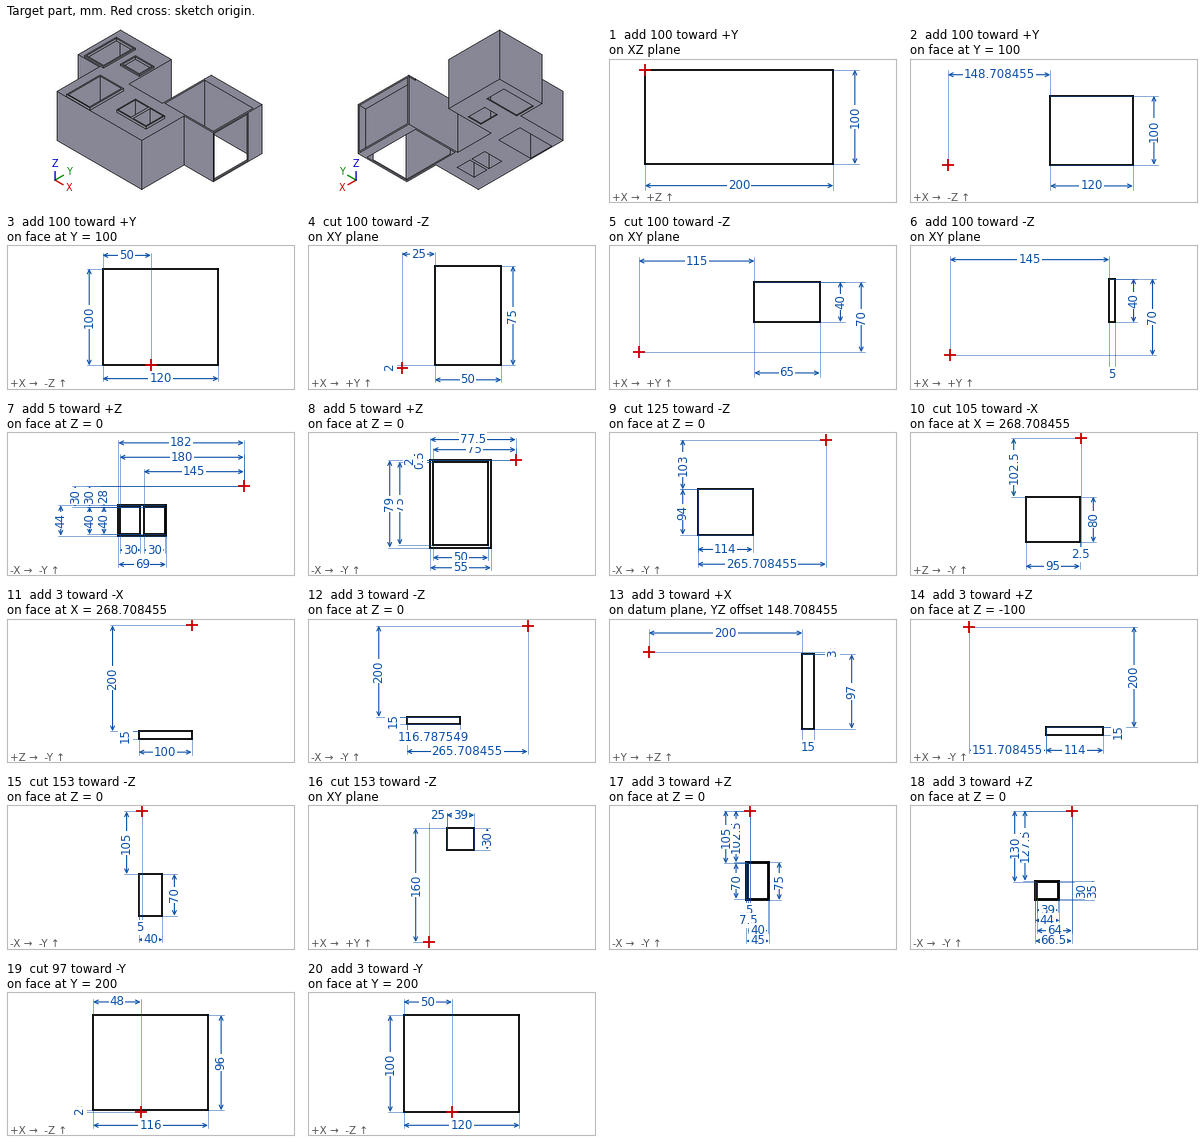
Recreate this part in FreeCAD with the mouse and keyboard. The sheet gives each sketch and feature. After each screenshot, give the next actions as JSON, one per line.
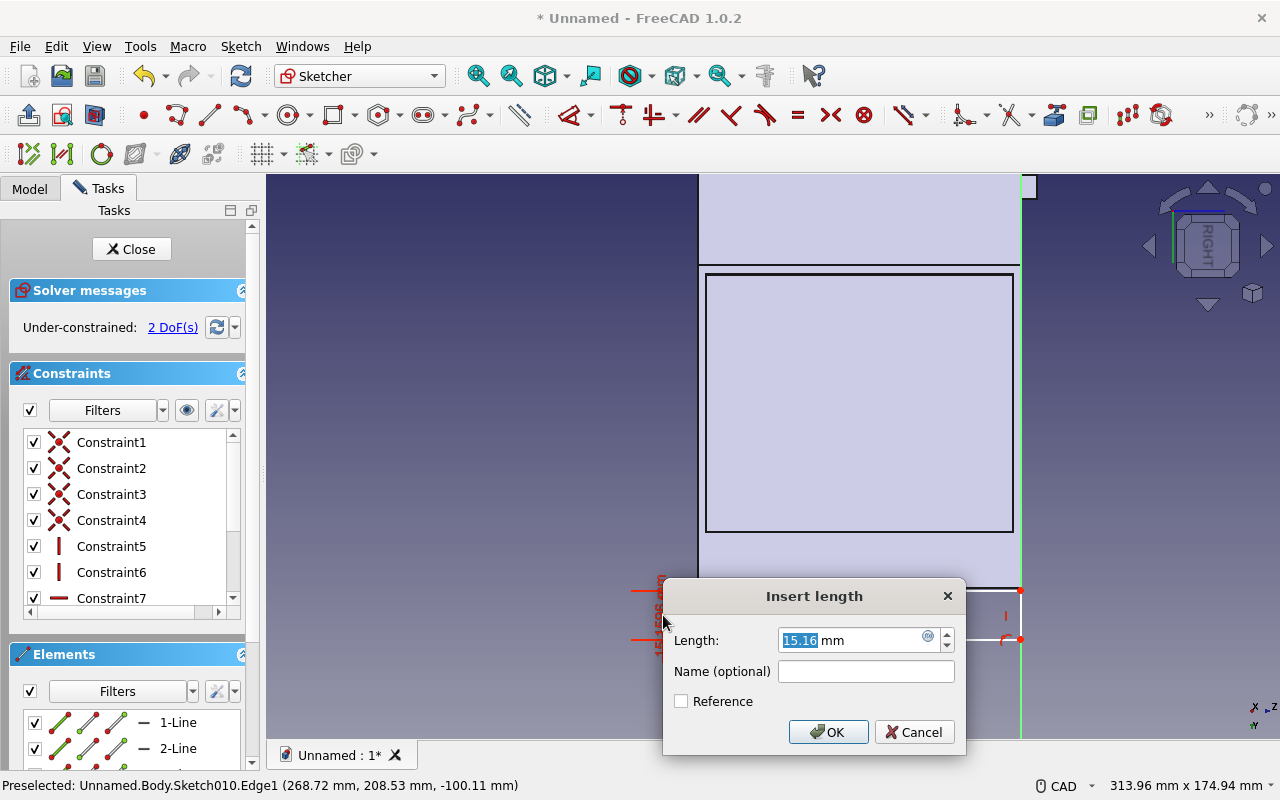
{"action": "type", "text": "15"}
{"action": "key", "text": "Return"}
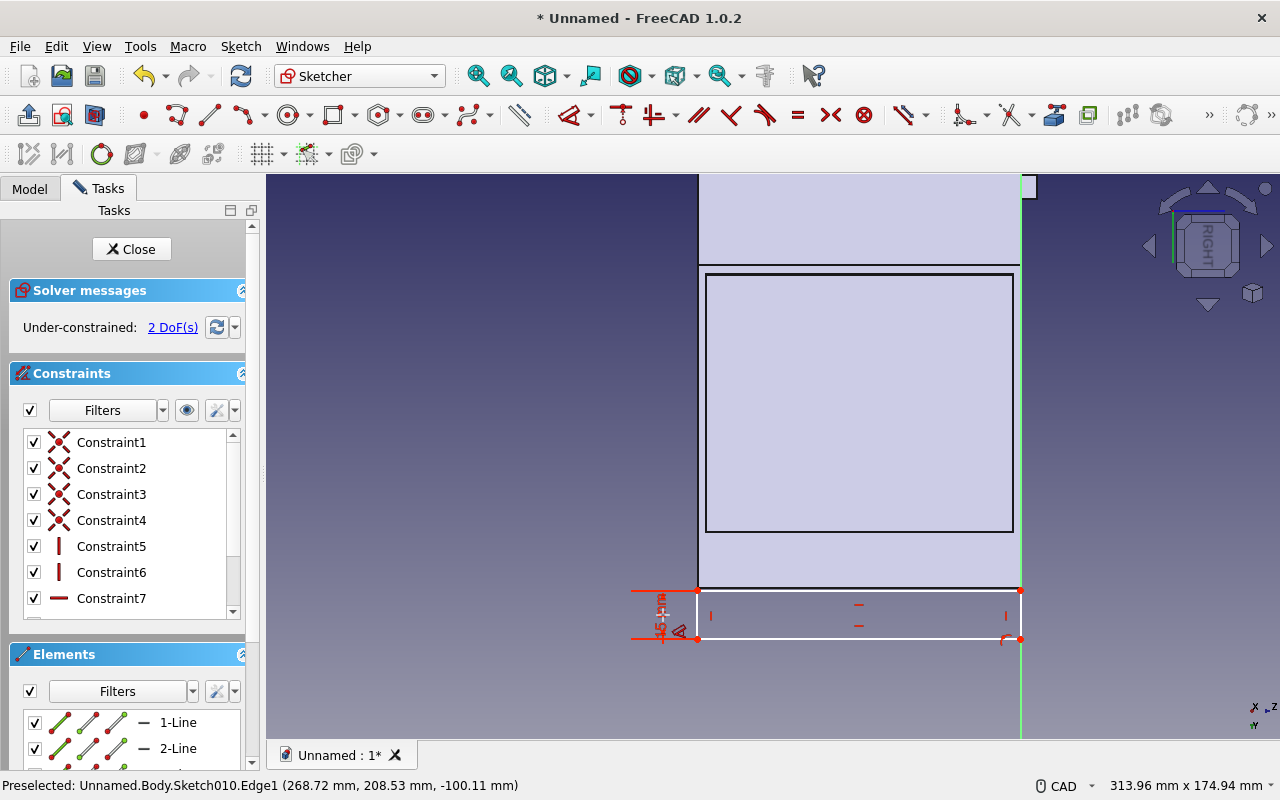
{"action": "left_click", "coordinate": [794, 639]}
{"action": "left_click", "coordinate": [859, 673]}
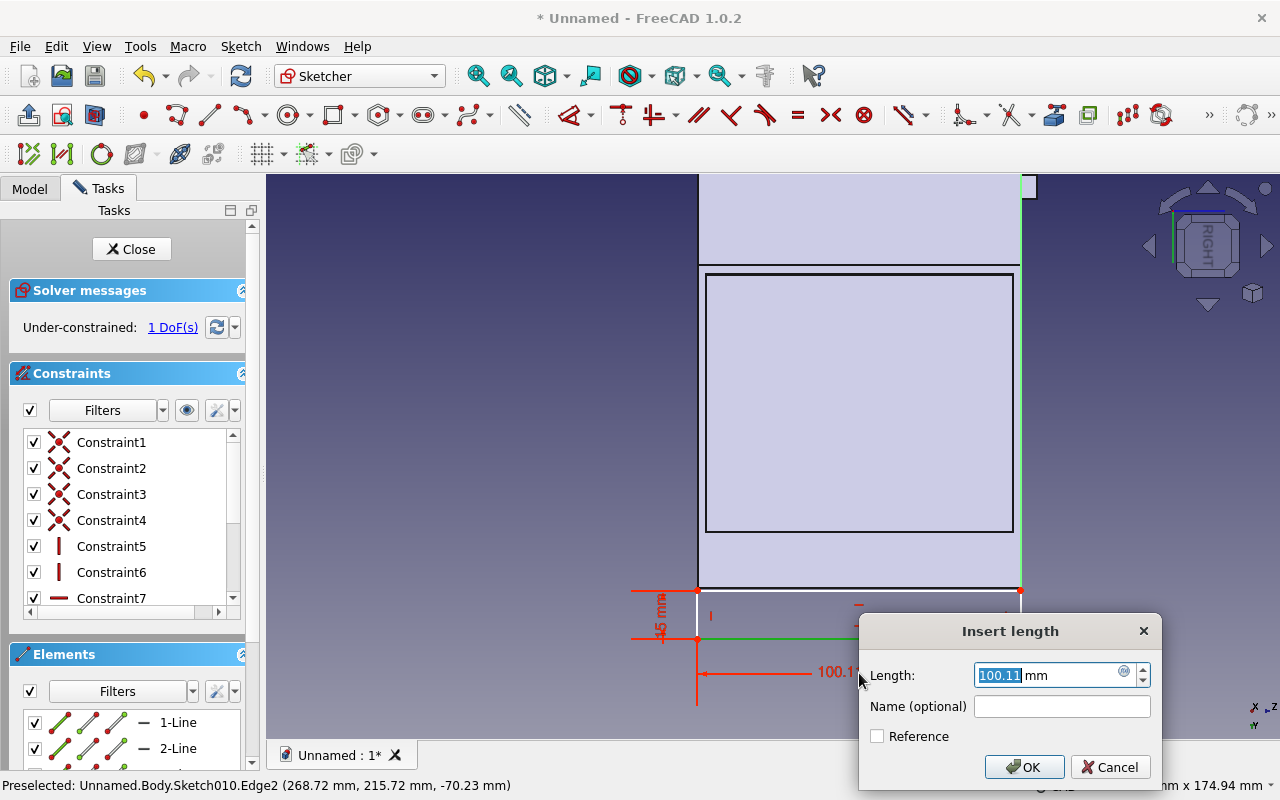
{"action": "type", "text": "100"}
{"action": "key", "text": "Return"}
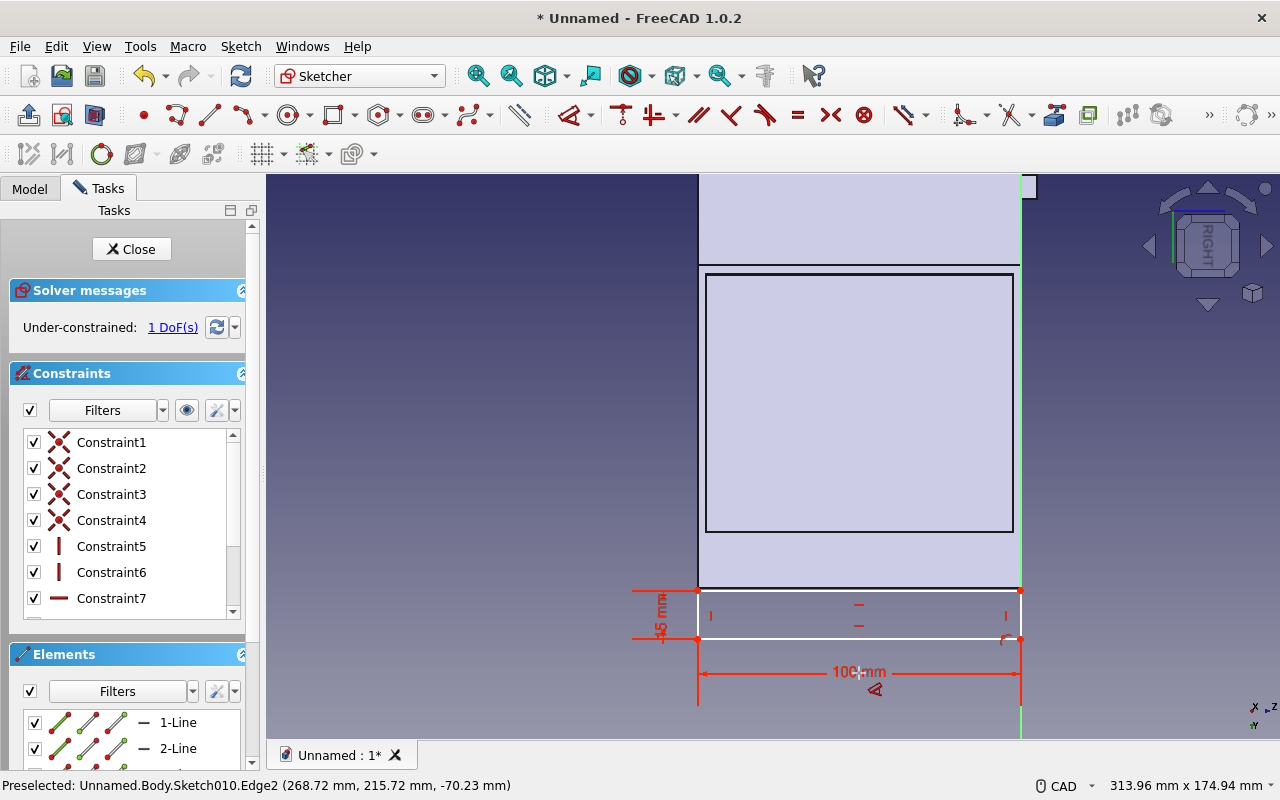
{"action": "left_click", "coordinate": [698, 591]}
{"action": "left_click", "coordinate": [1055, 396]}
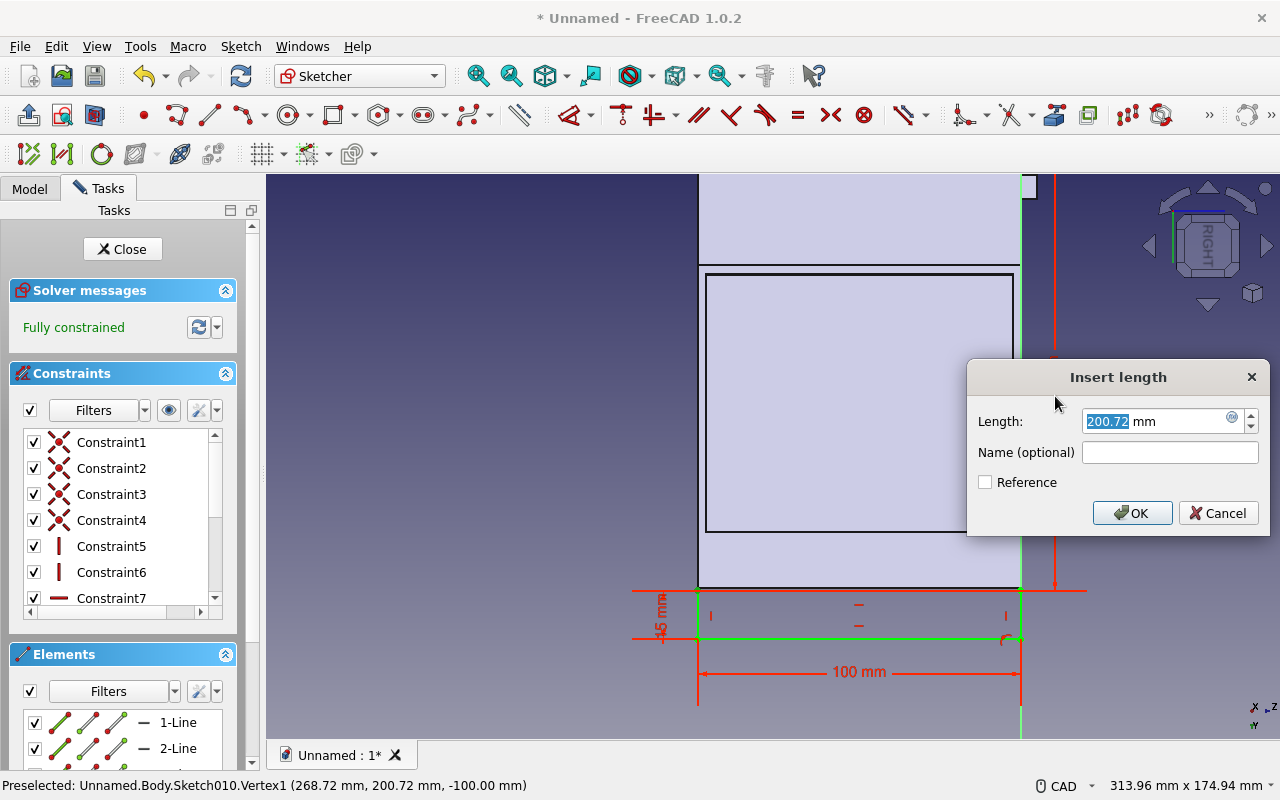
{"action": "type", "text": "200"}
{"action": "key", "text": "Return"}
{"action": "key", "text": "Escape"}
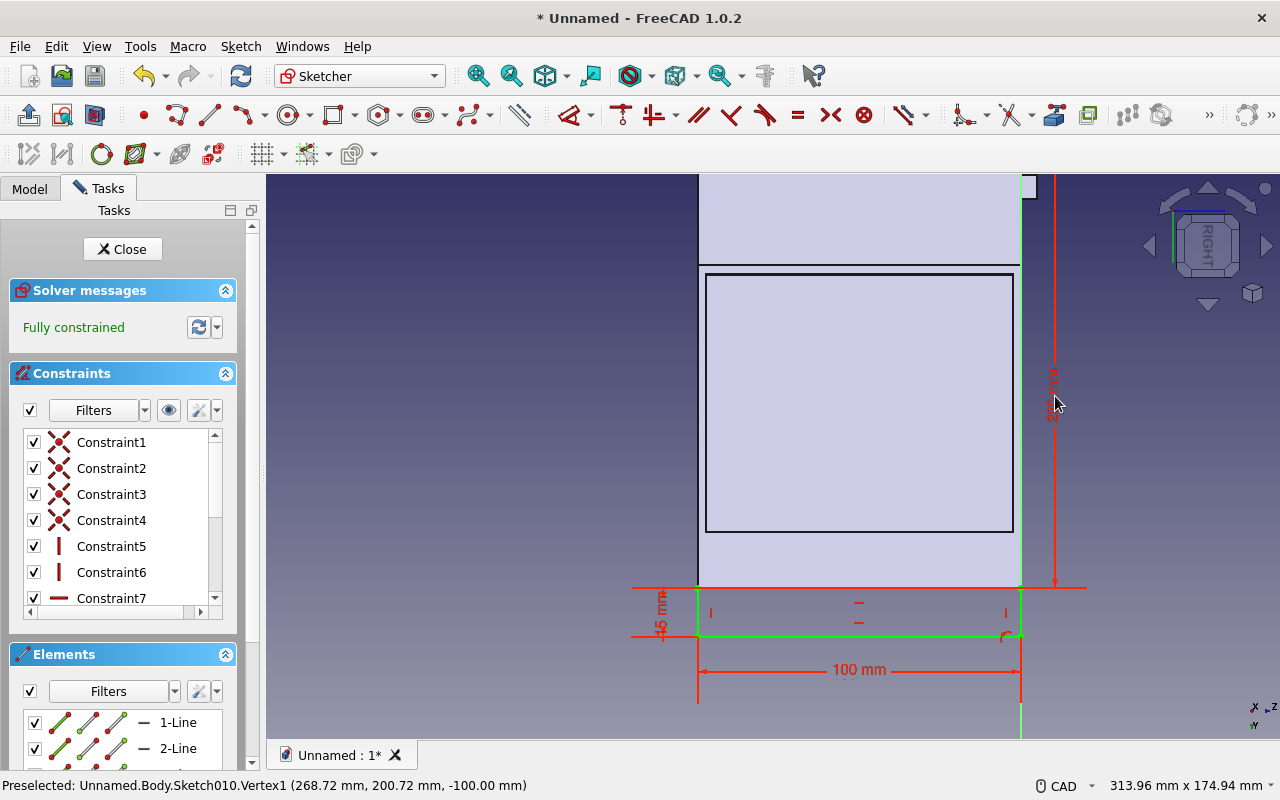
{"action": "left_click", "coordinate": [123, 249]}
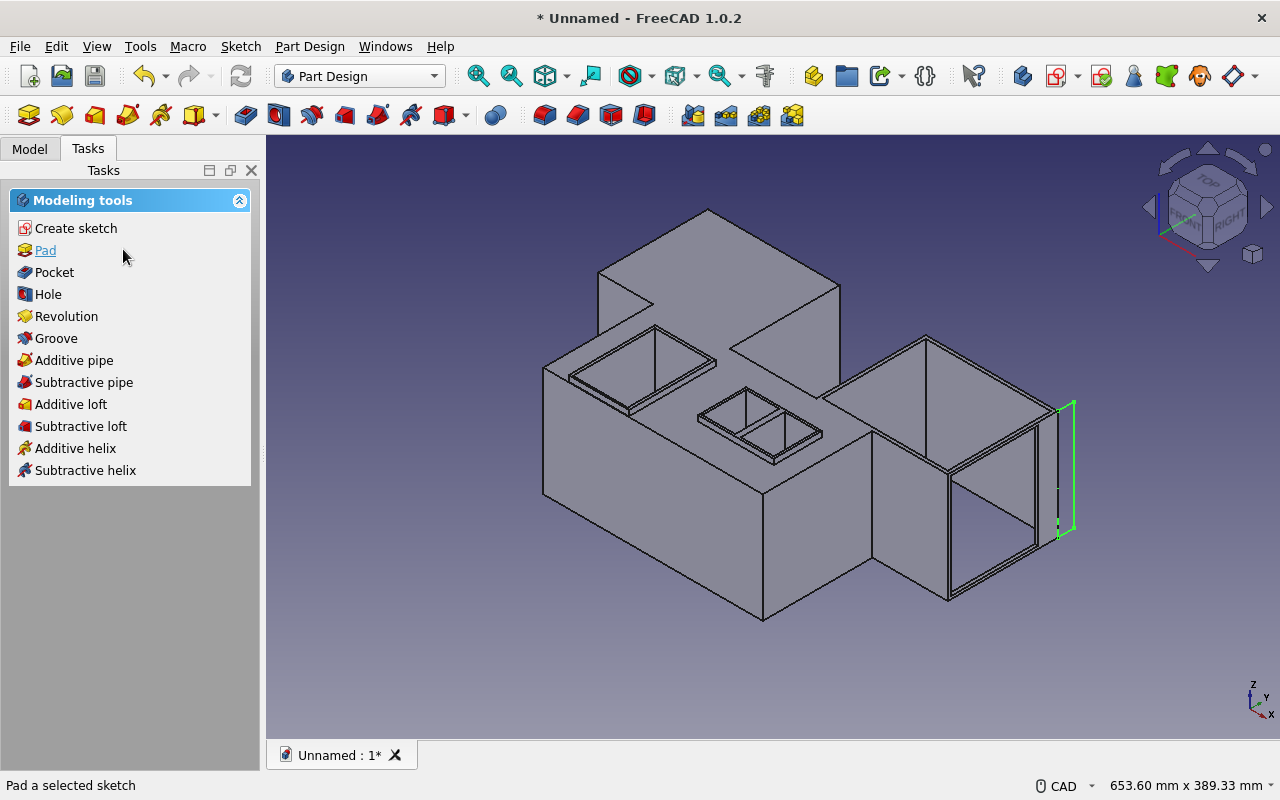
{"action": "left_click", "coordinate": [29, 116]}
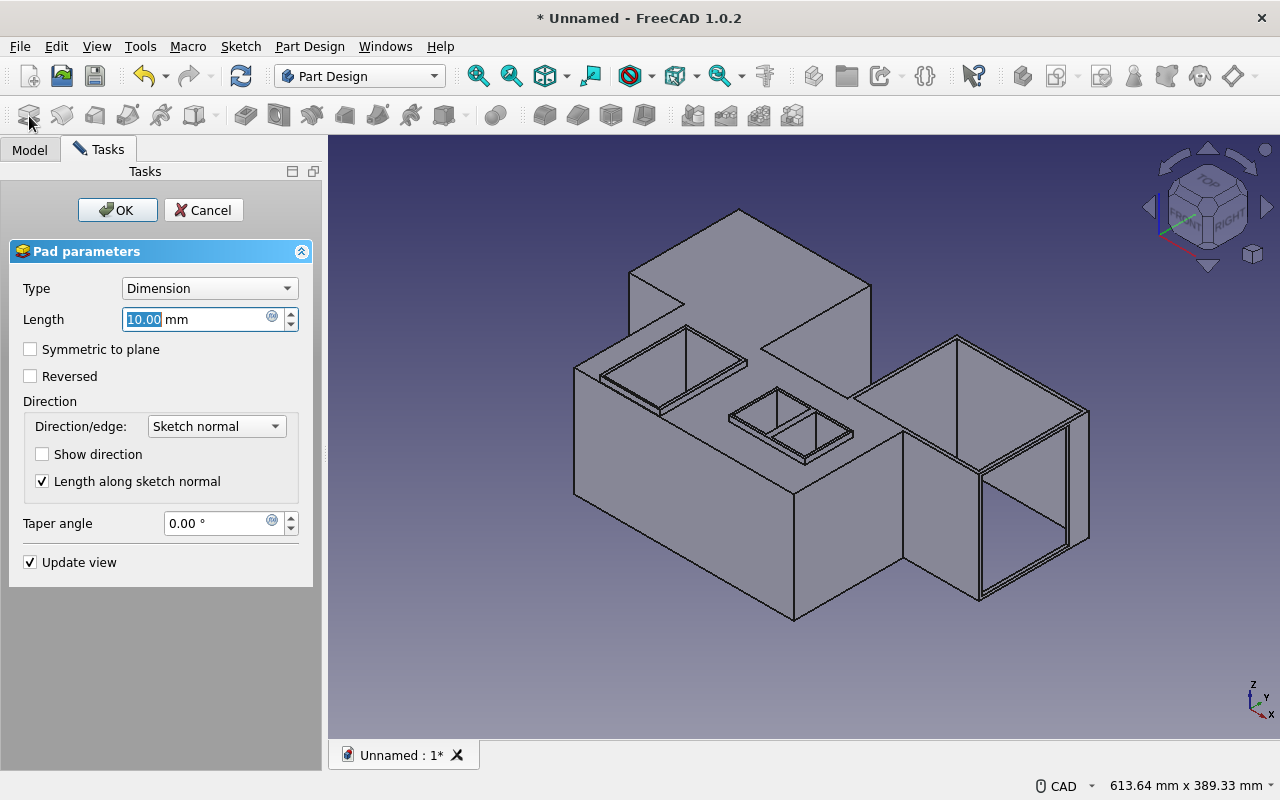
{"action": "type", "text": "3"}
{"action": "key", "text": "Tab"}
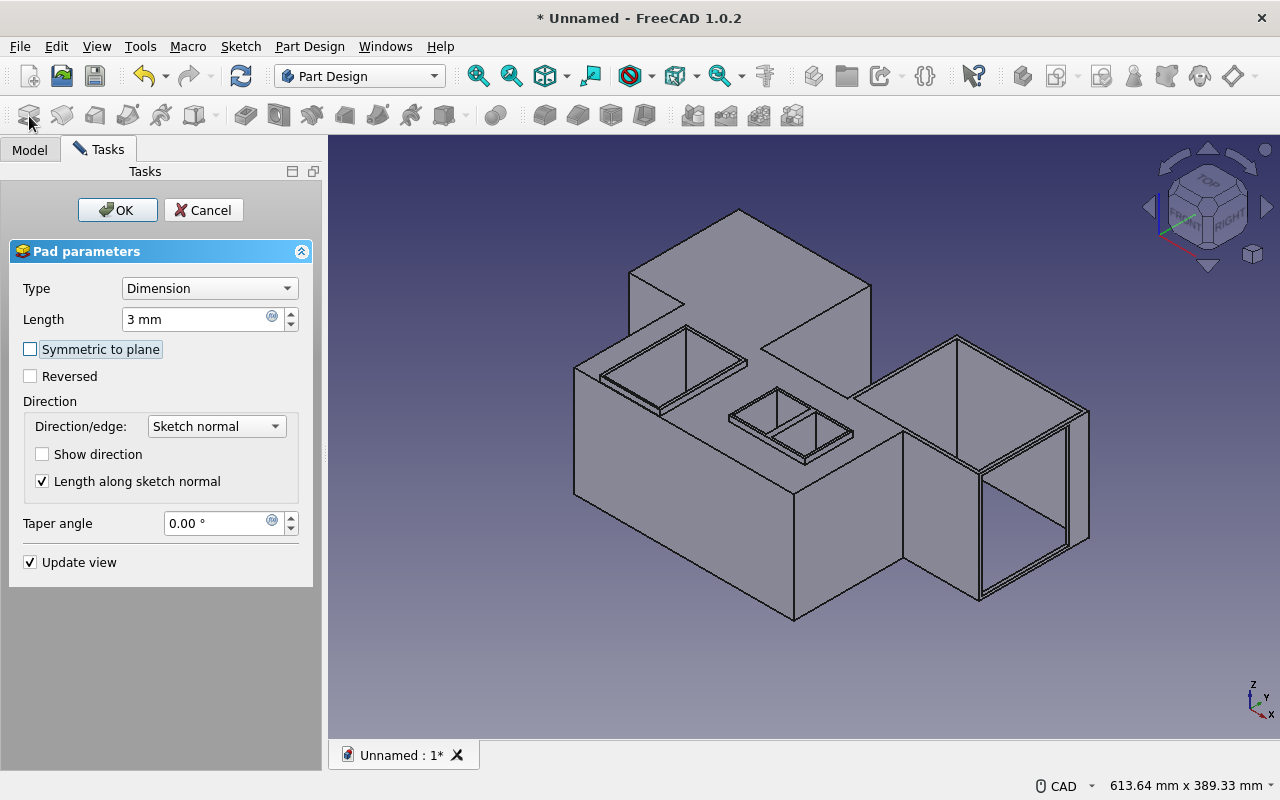
{"action": "left_click", "coordinate": [31, 376]}